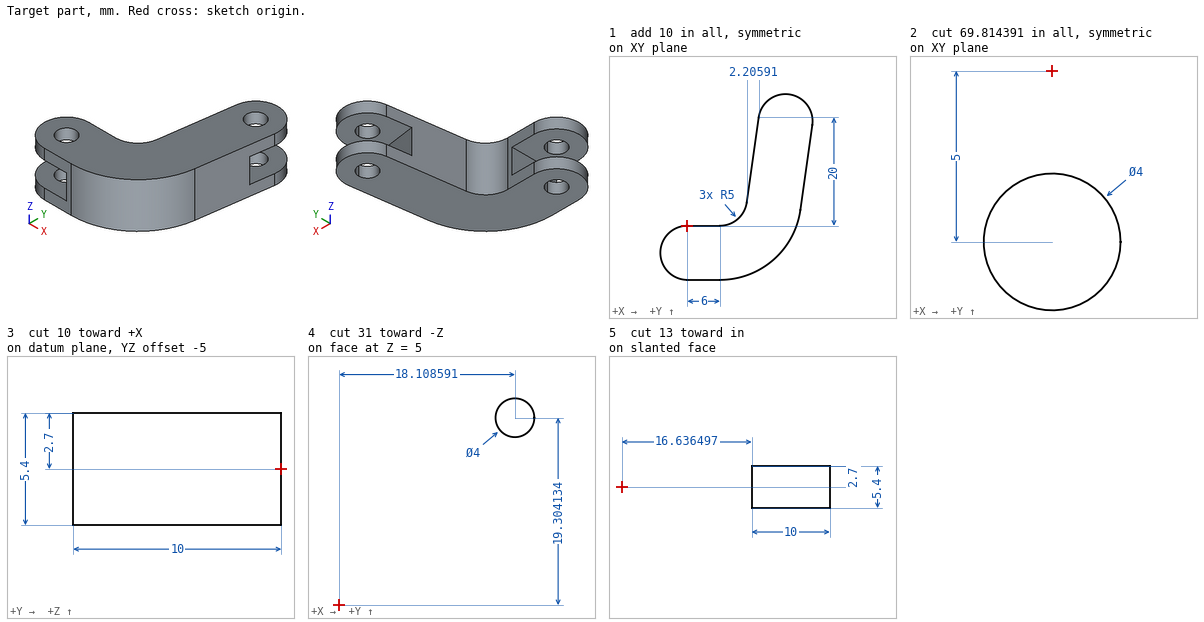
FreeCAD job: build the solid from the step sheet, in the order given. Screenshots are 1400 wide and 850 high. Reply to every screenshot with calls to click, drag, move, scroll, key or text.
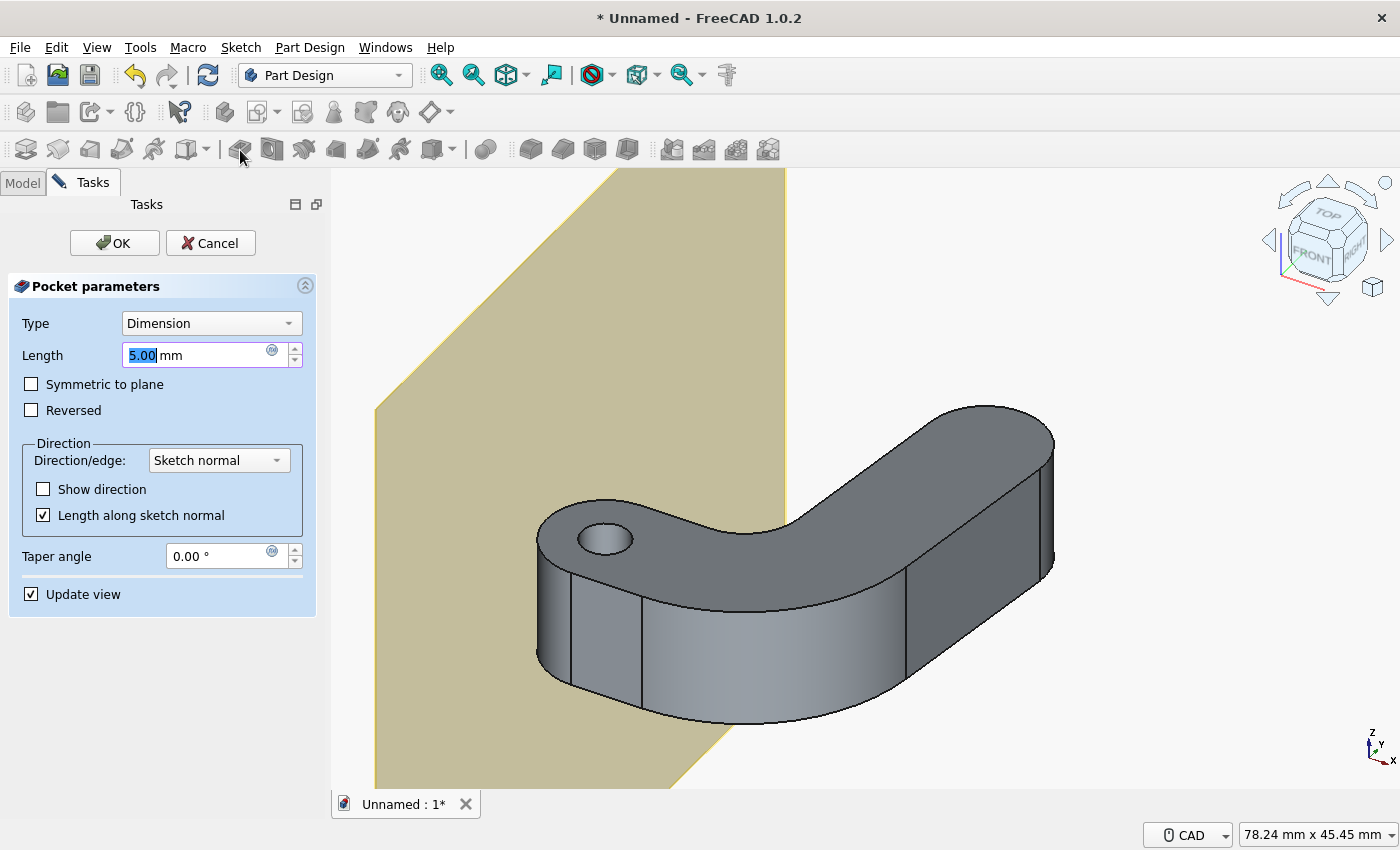
text(10)
key(Tab)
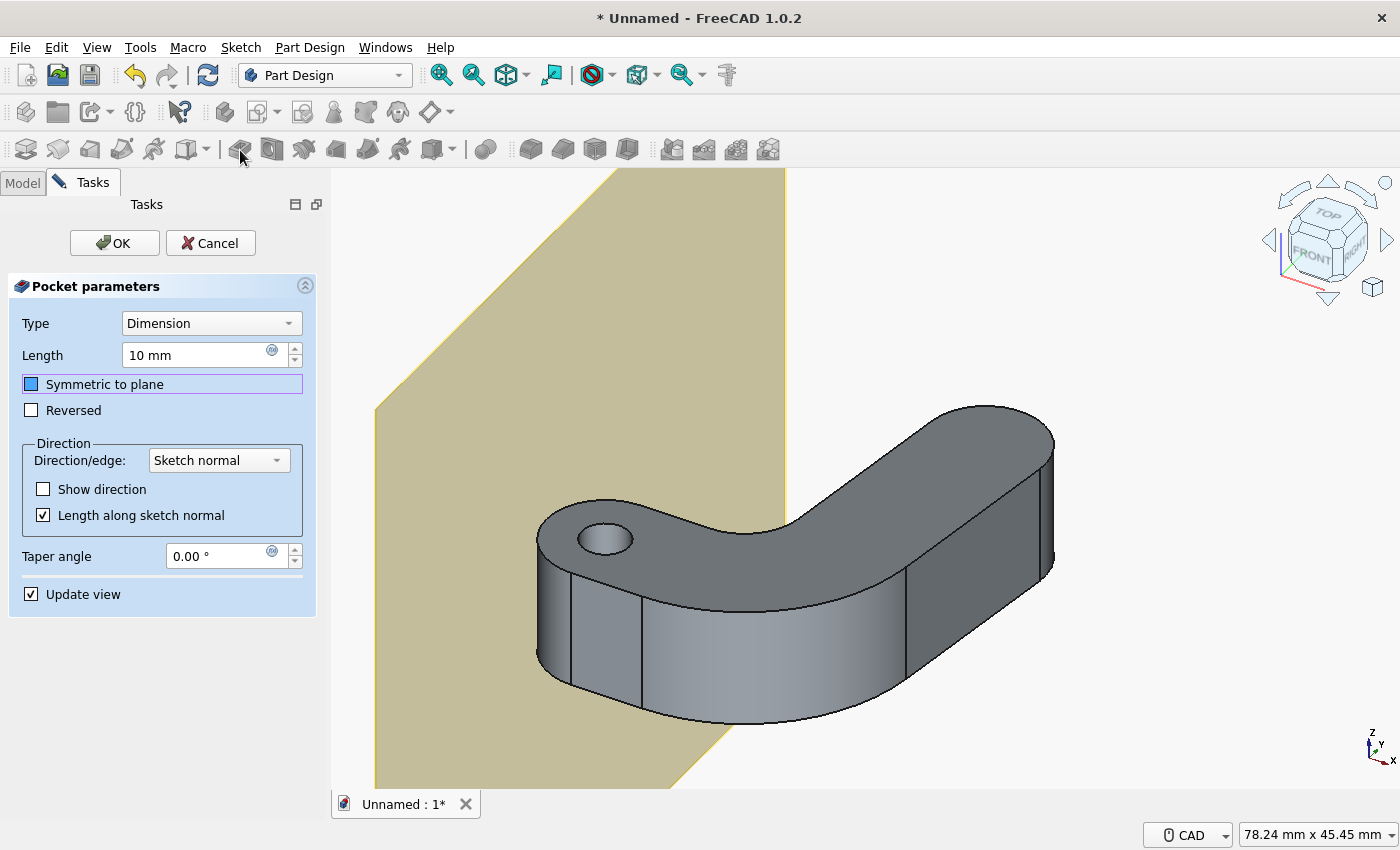
click(30, 410)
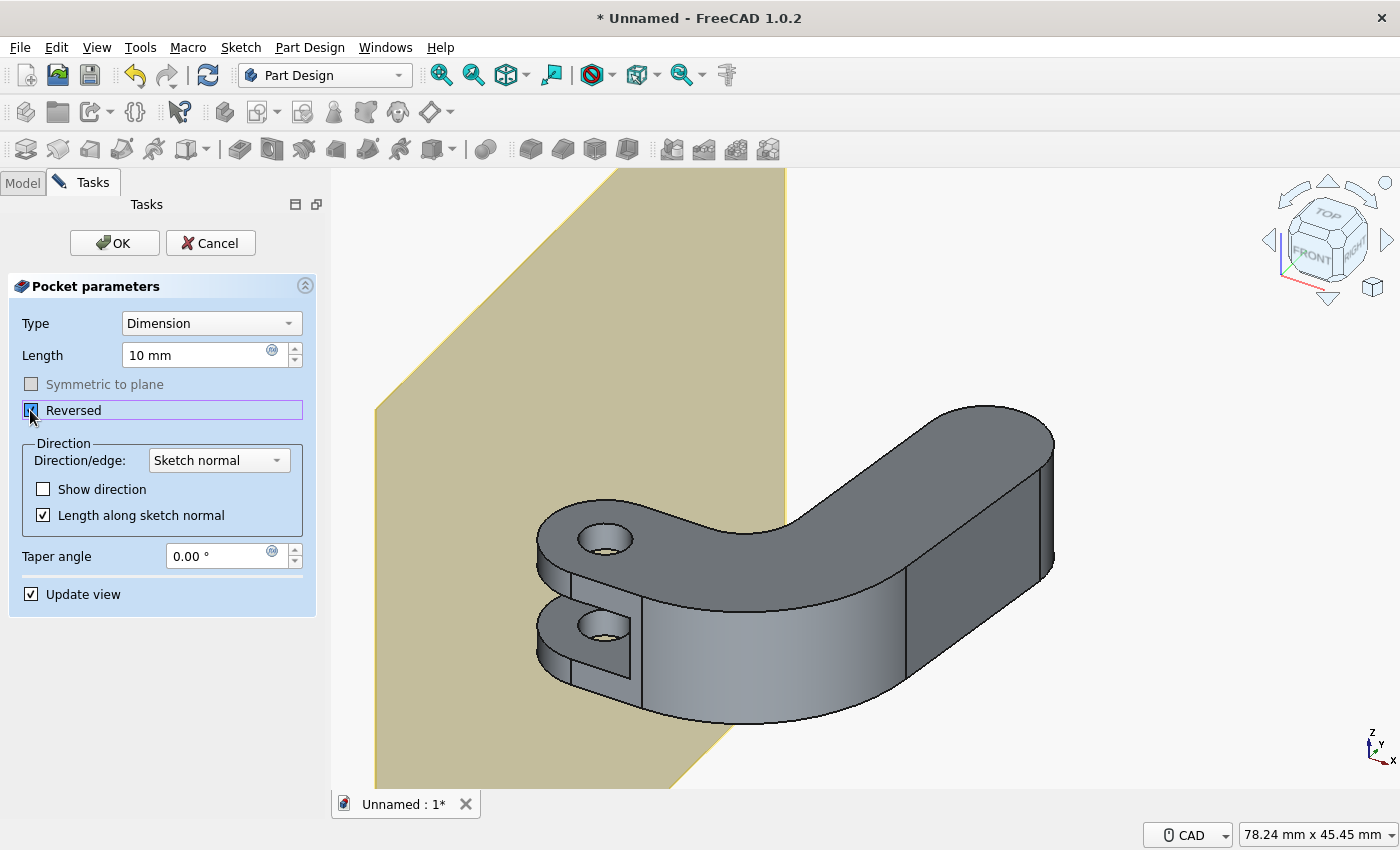
click(115, 243)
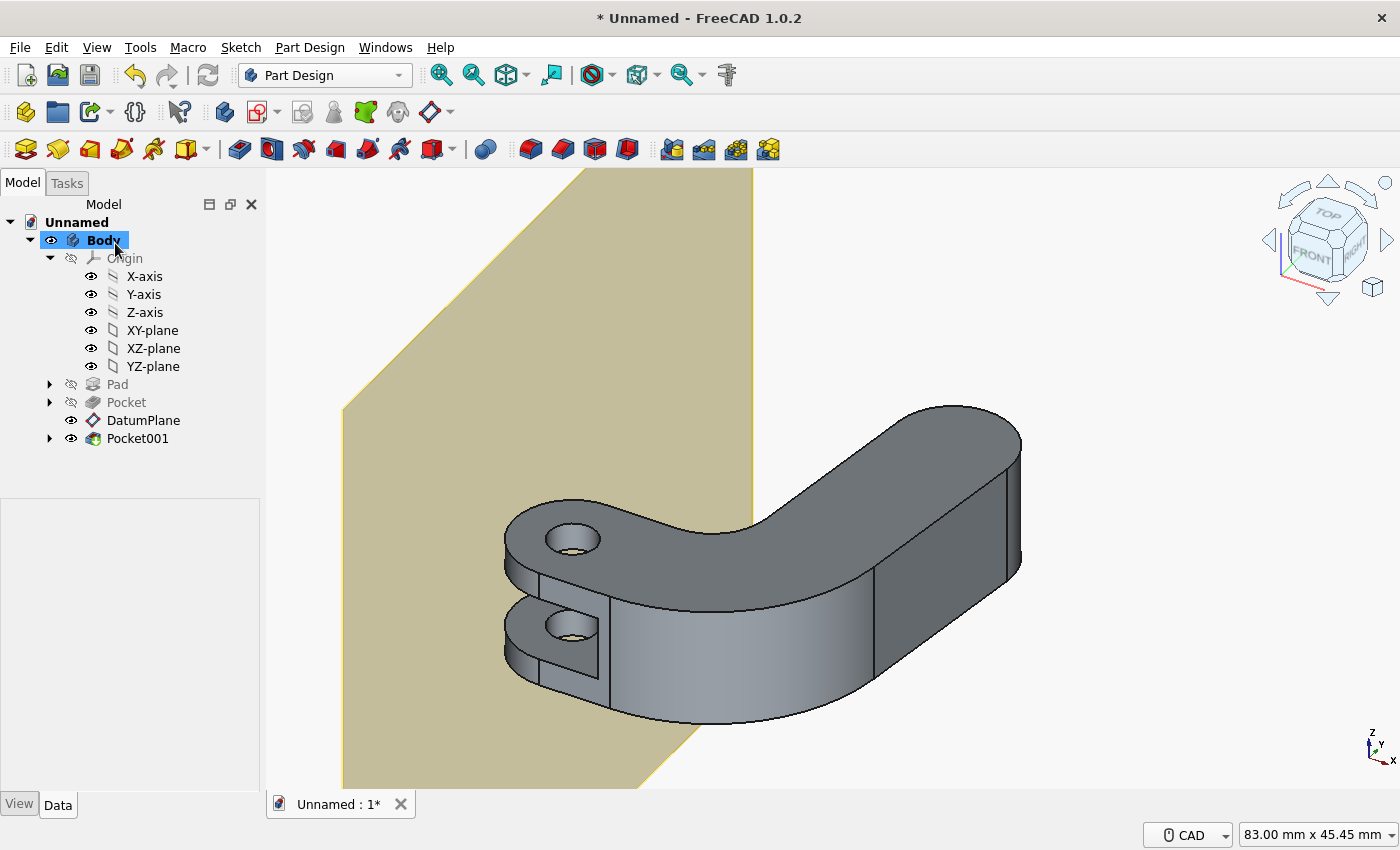
click(116, 420)
key(space)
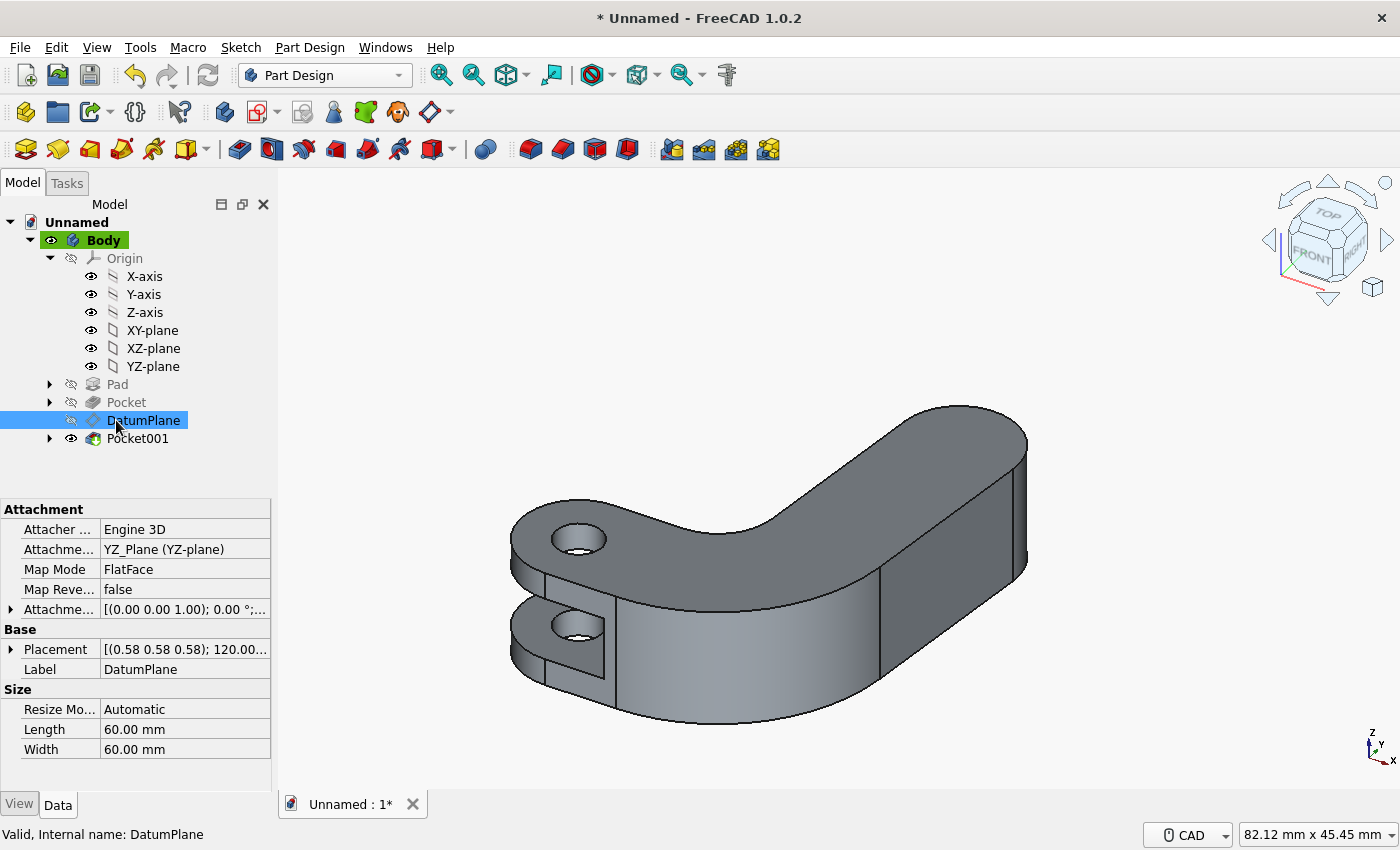
click(898, 489)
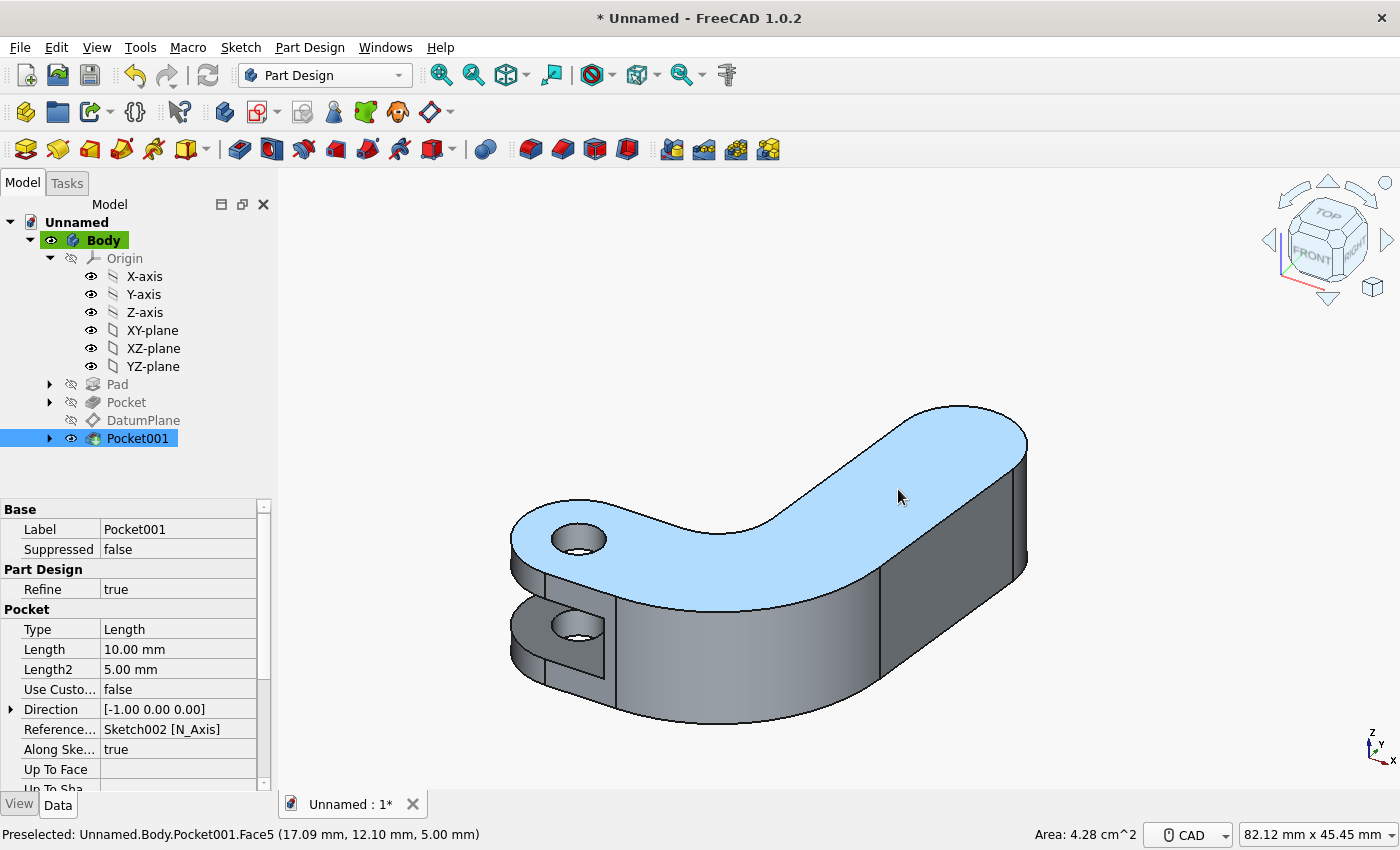
click(258, 112)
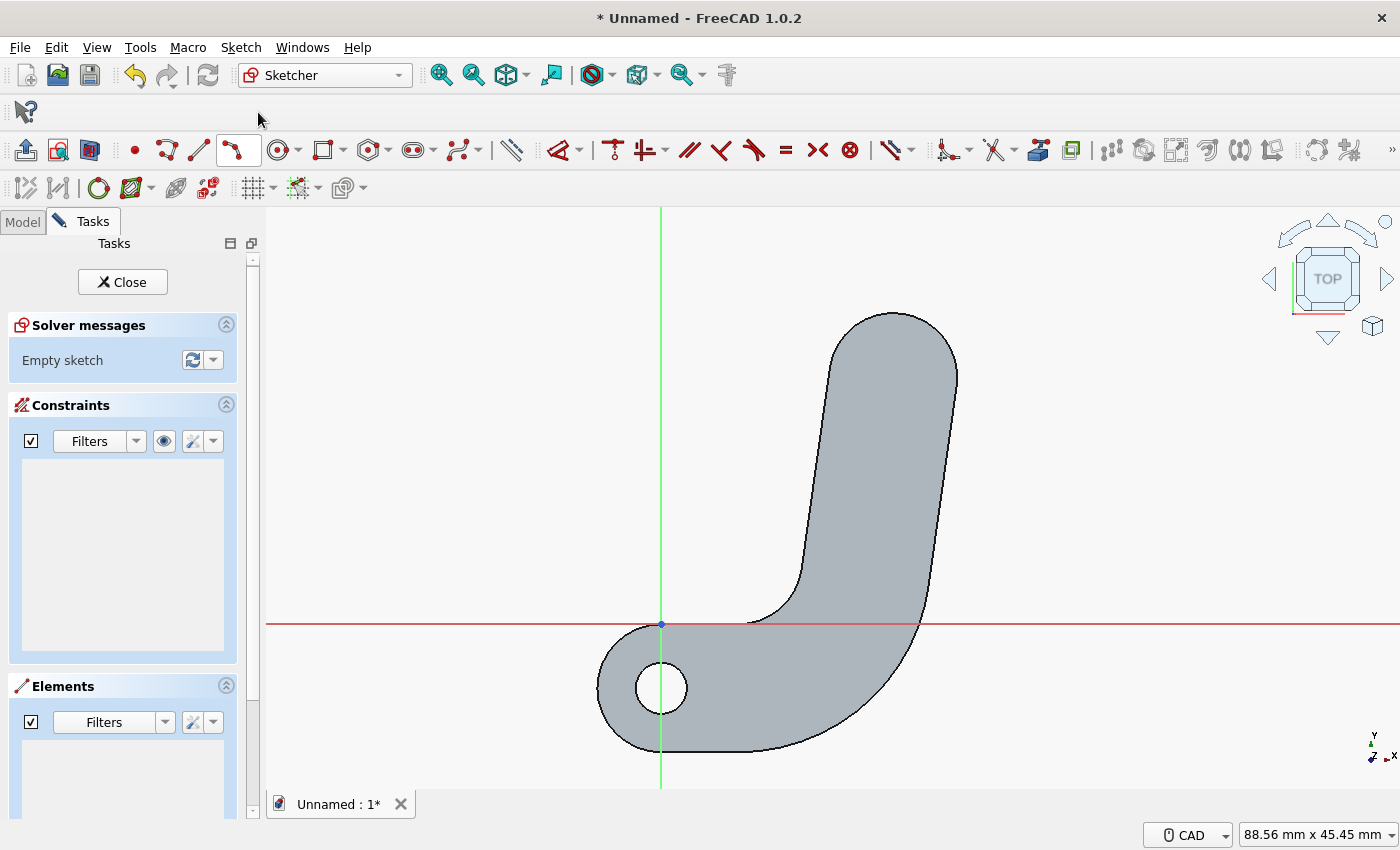
scroll(913, 358, up, 10)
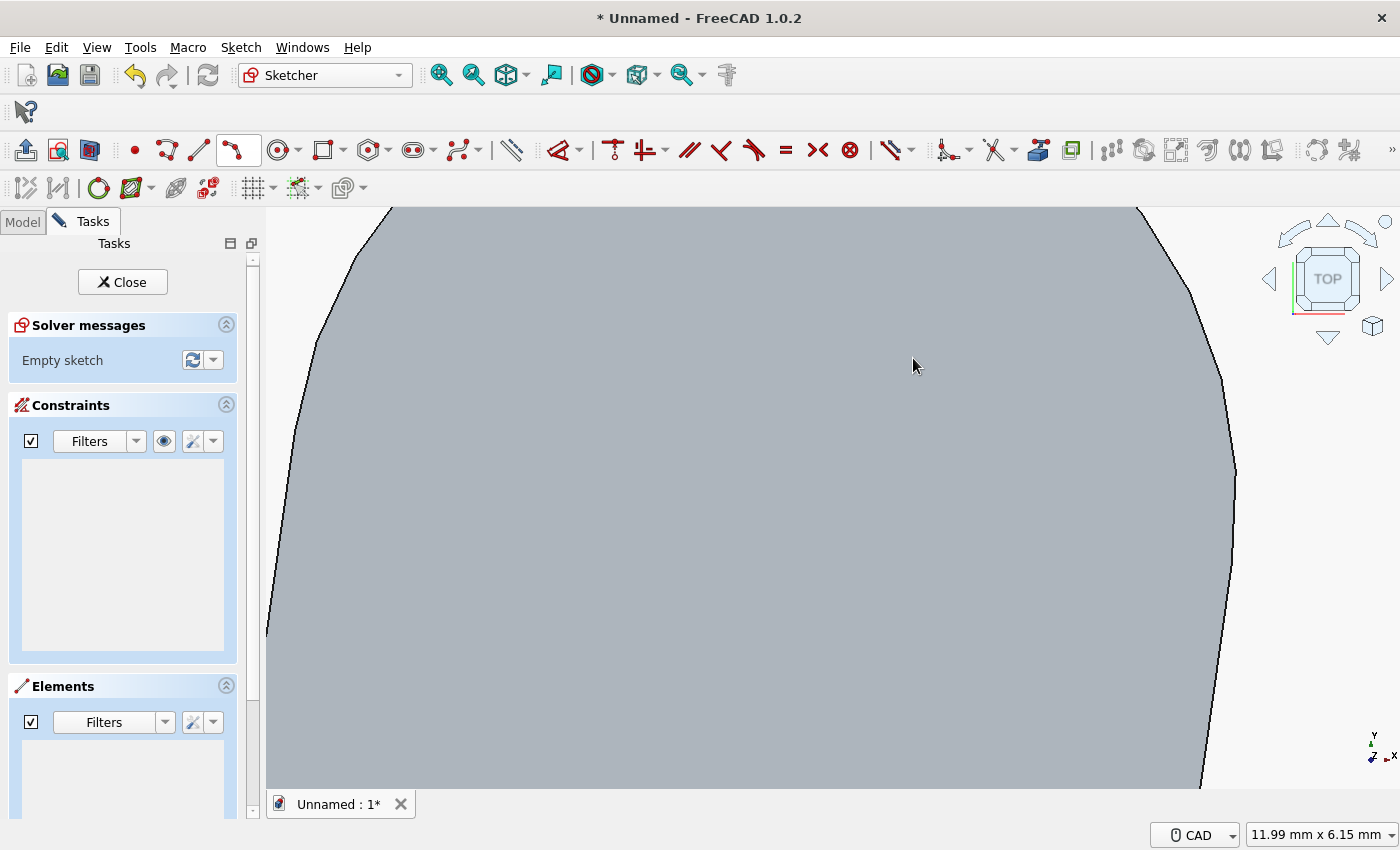
key(g)
key(c)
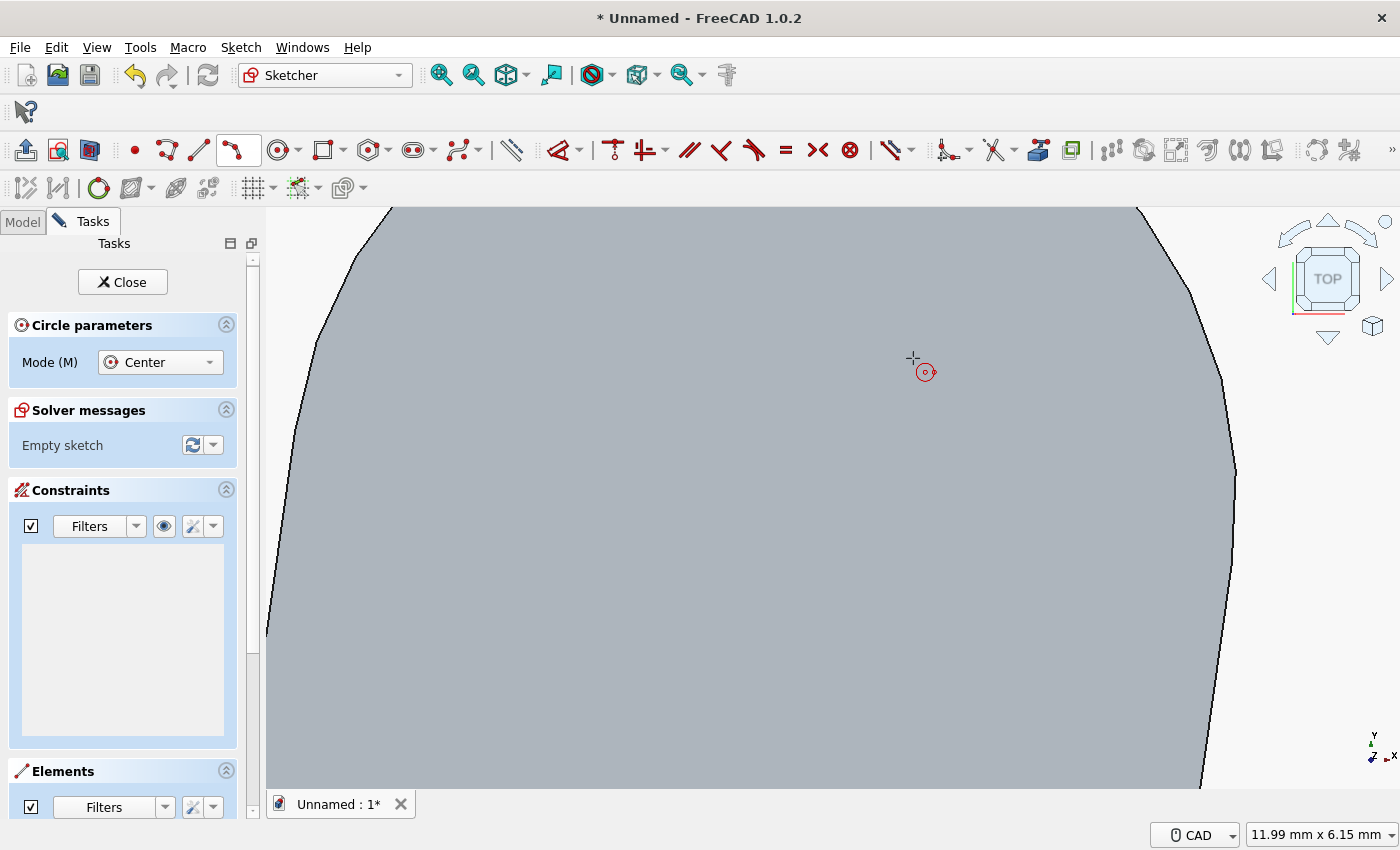
click(763, 497)
click(897, 363)
key(Escape)